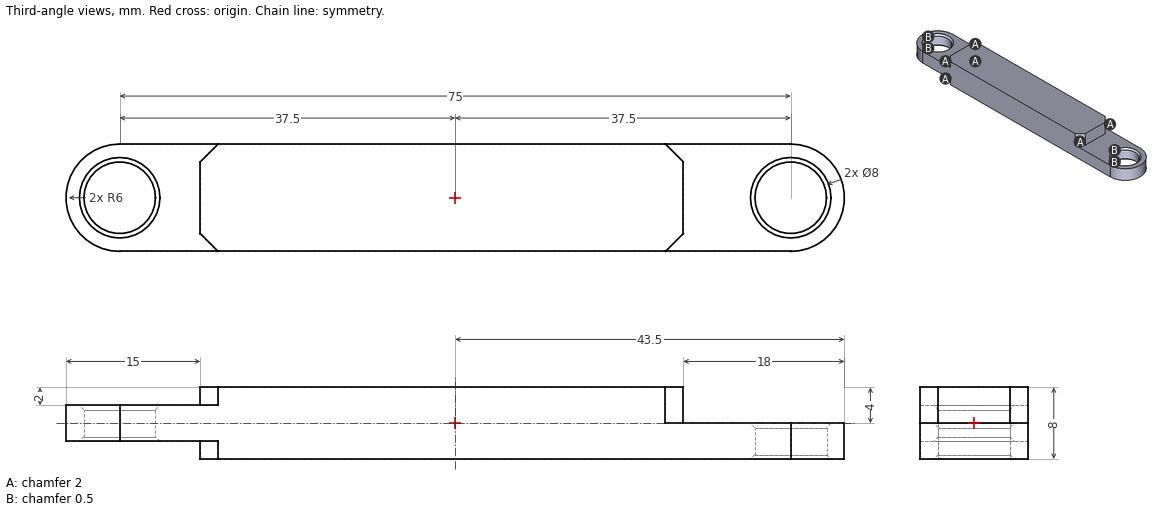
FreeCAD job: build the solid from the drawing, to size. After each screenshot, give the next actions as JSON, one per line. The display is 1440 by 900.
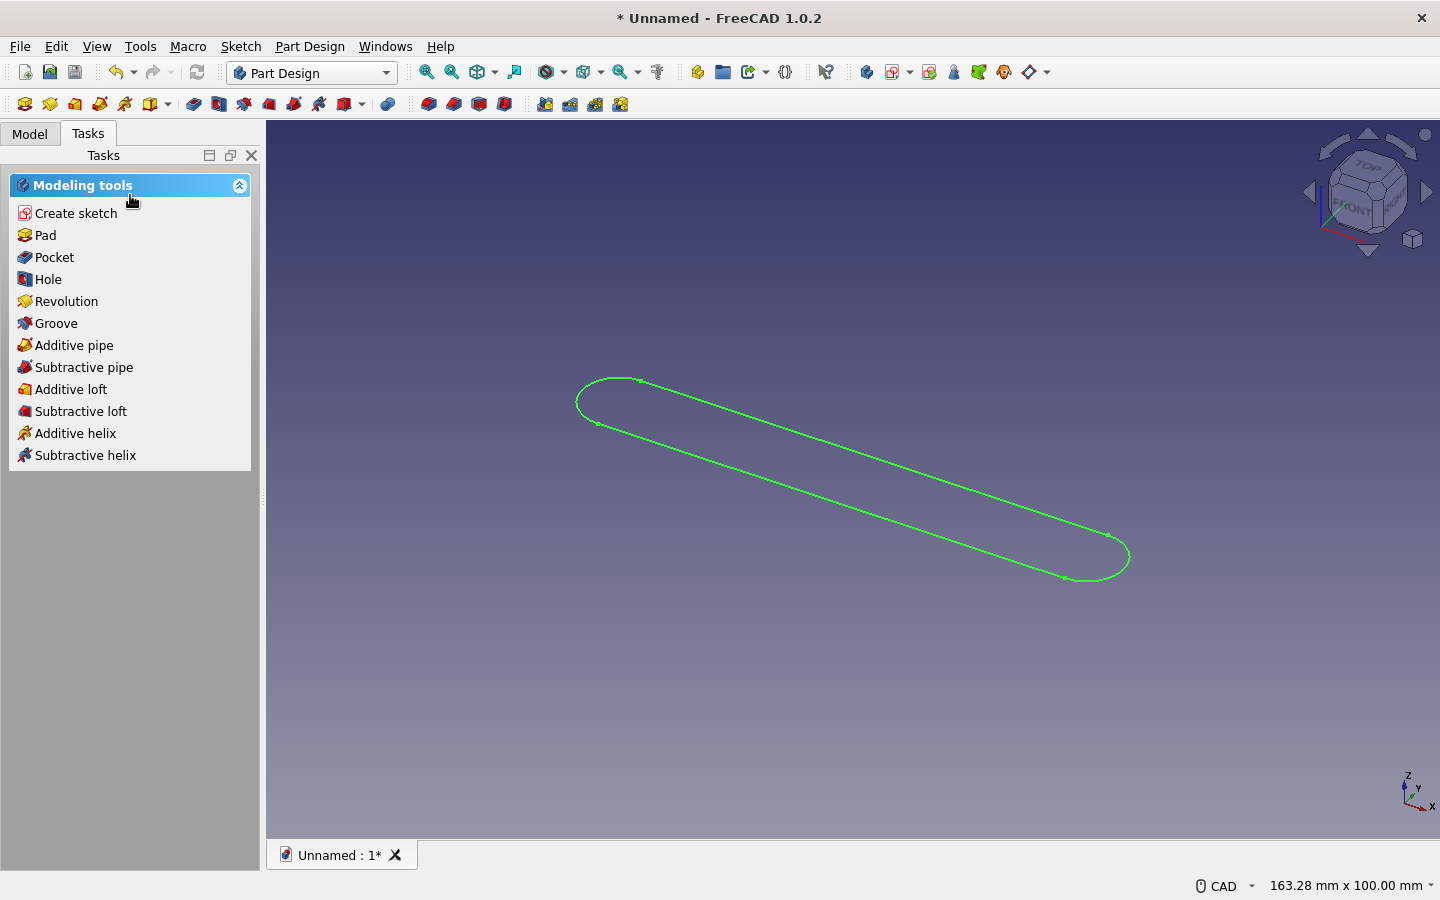
{"action": "left_click", "coordinate": [25, 104]}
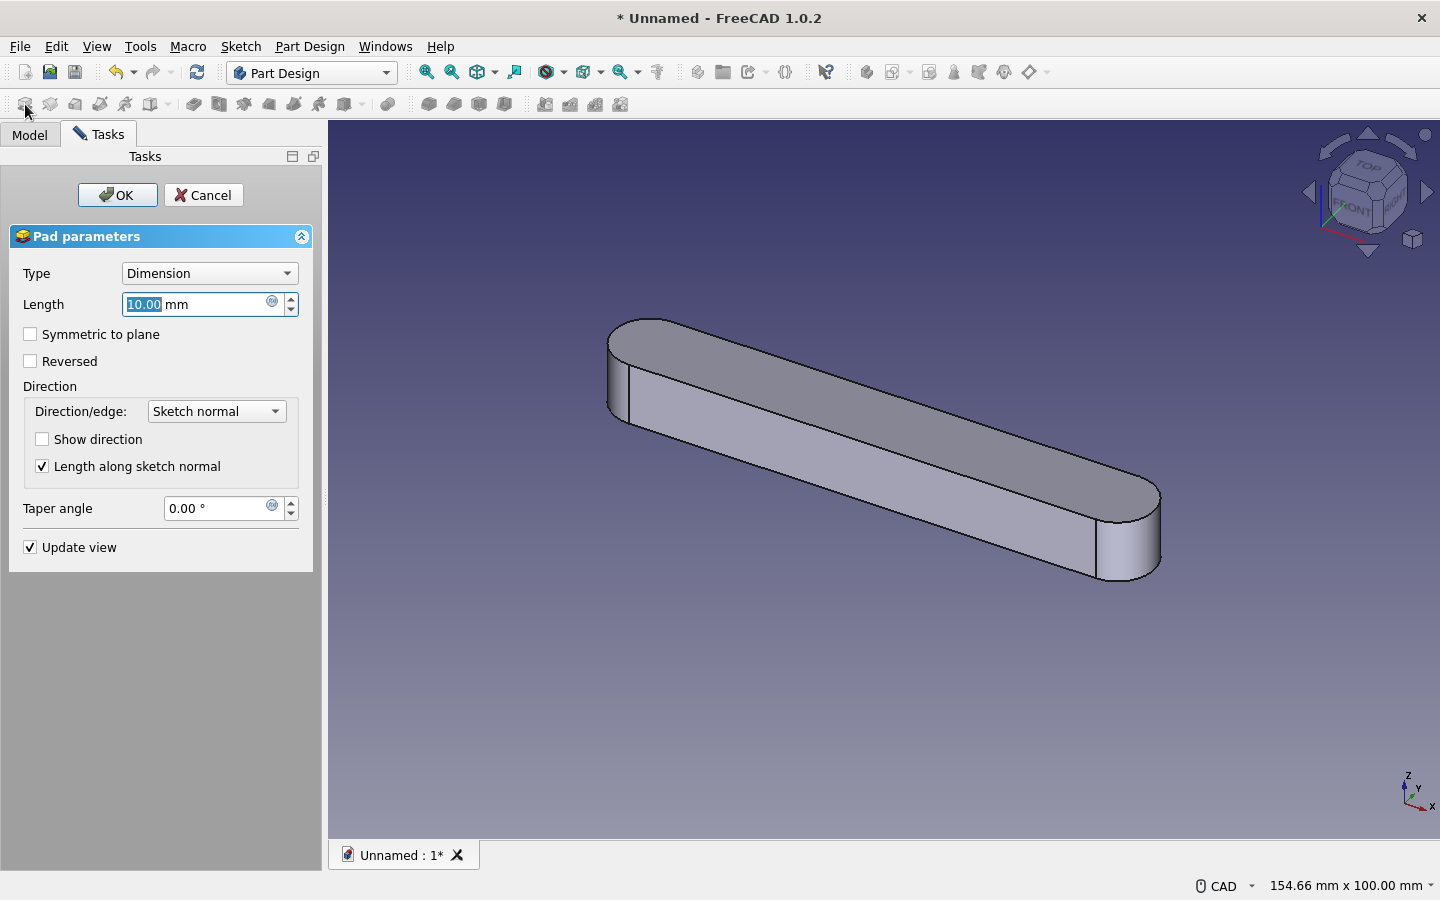
{"action": "type", "text": "8"}
{"action": "key", "text": "Tab"}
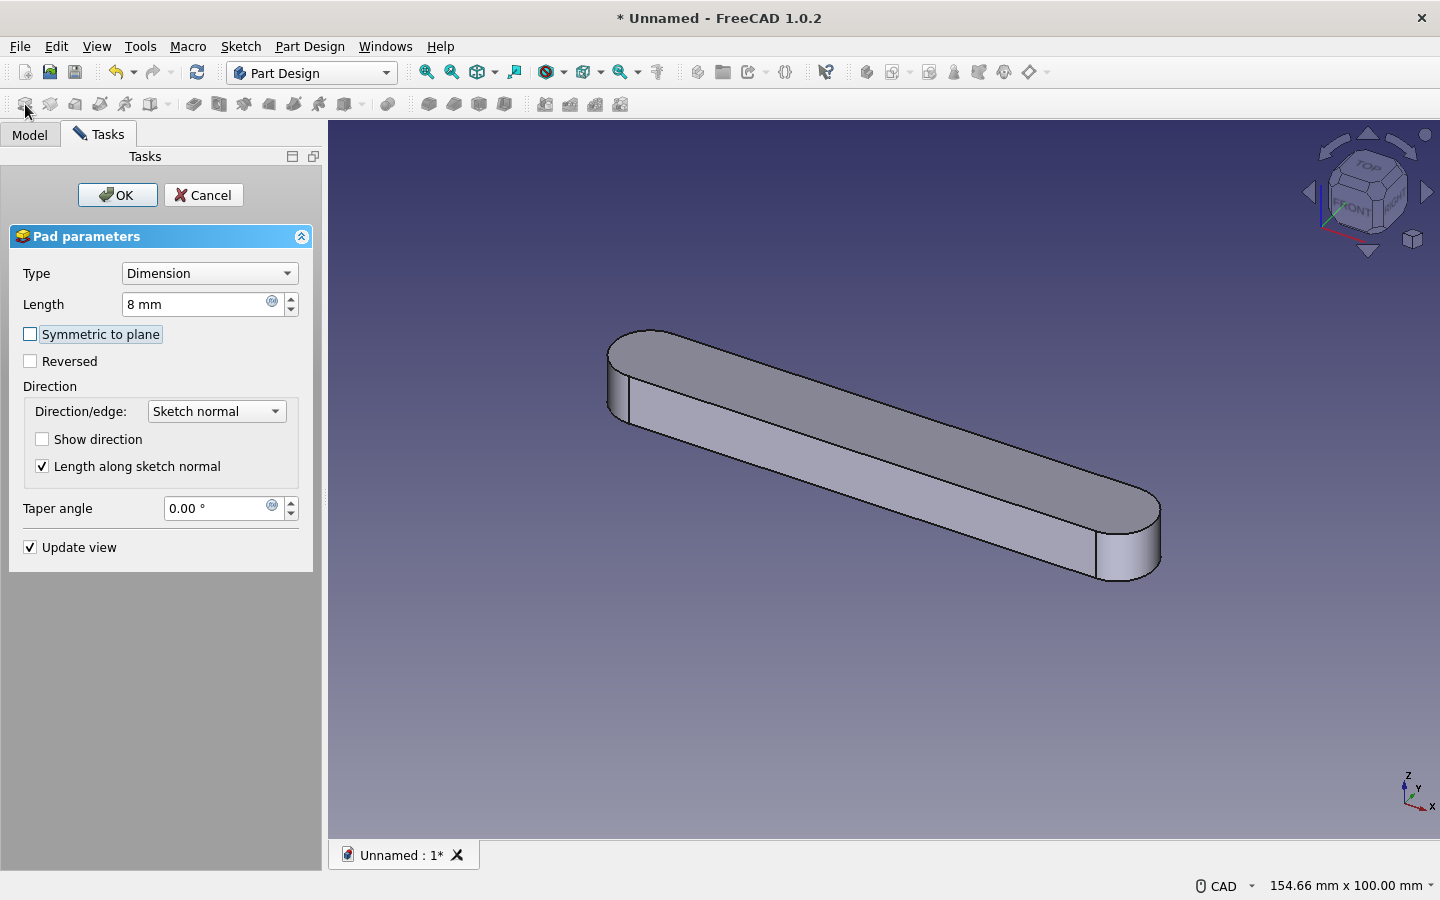
{"action": "left_click", "coordinate": [31, 334]}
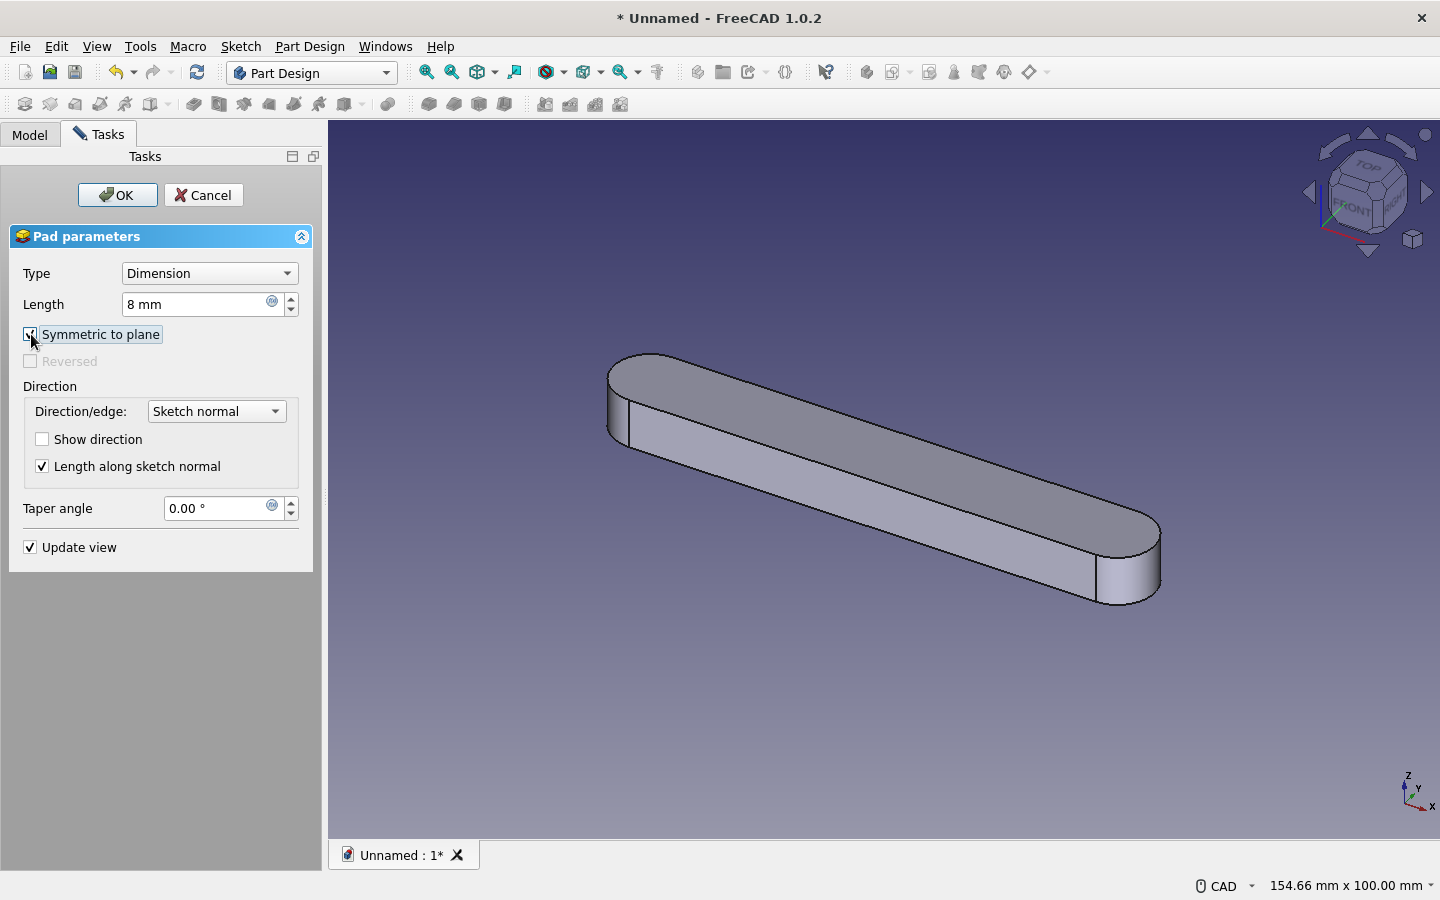
{"action": "left_click", "coordinate": [118, 195]}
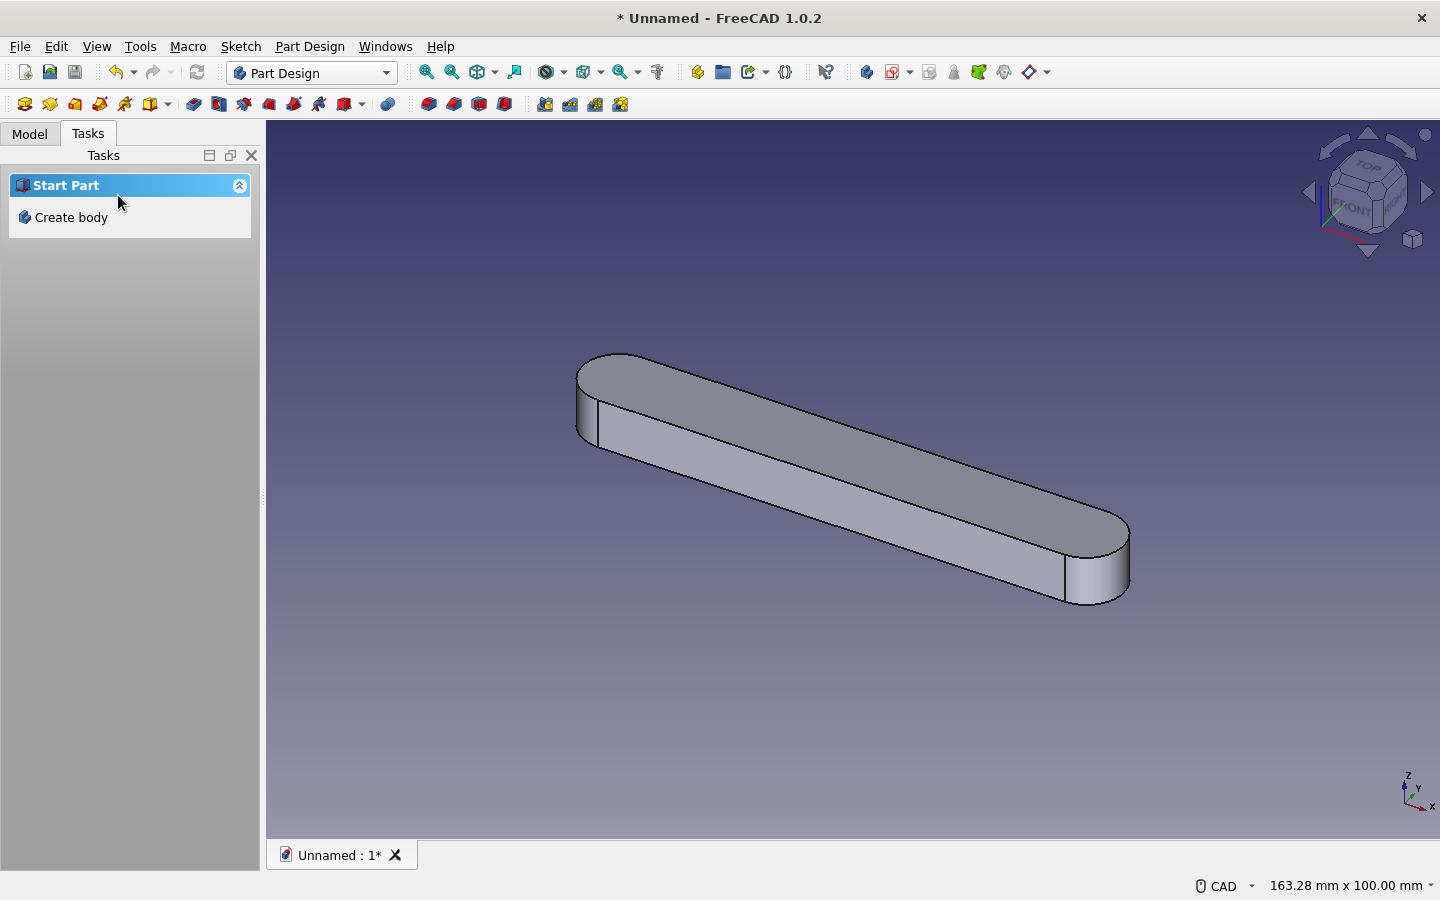
{"action": "left_click", "coordinate": [1085, 532]}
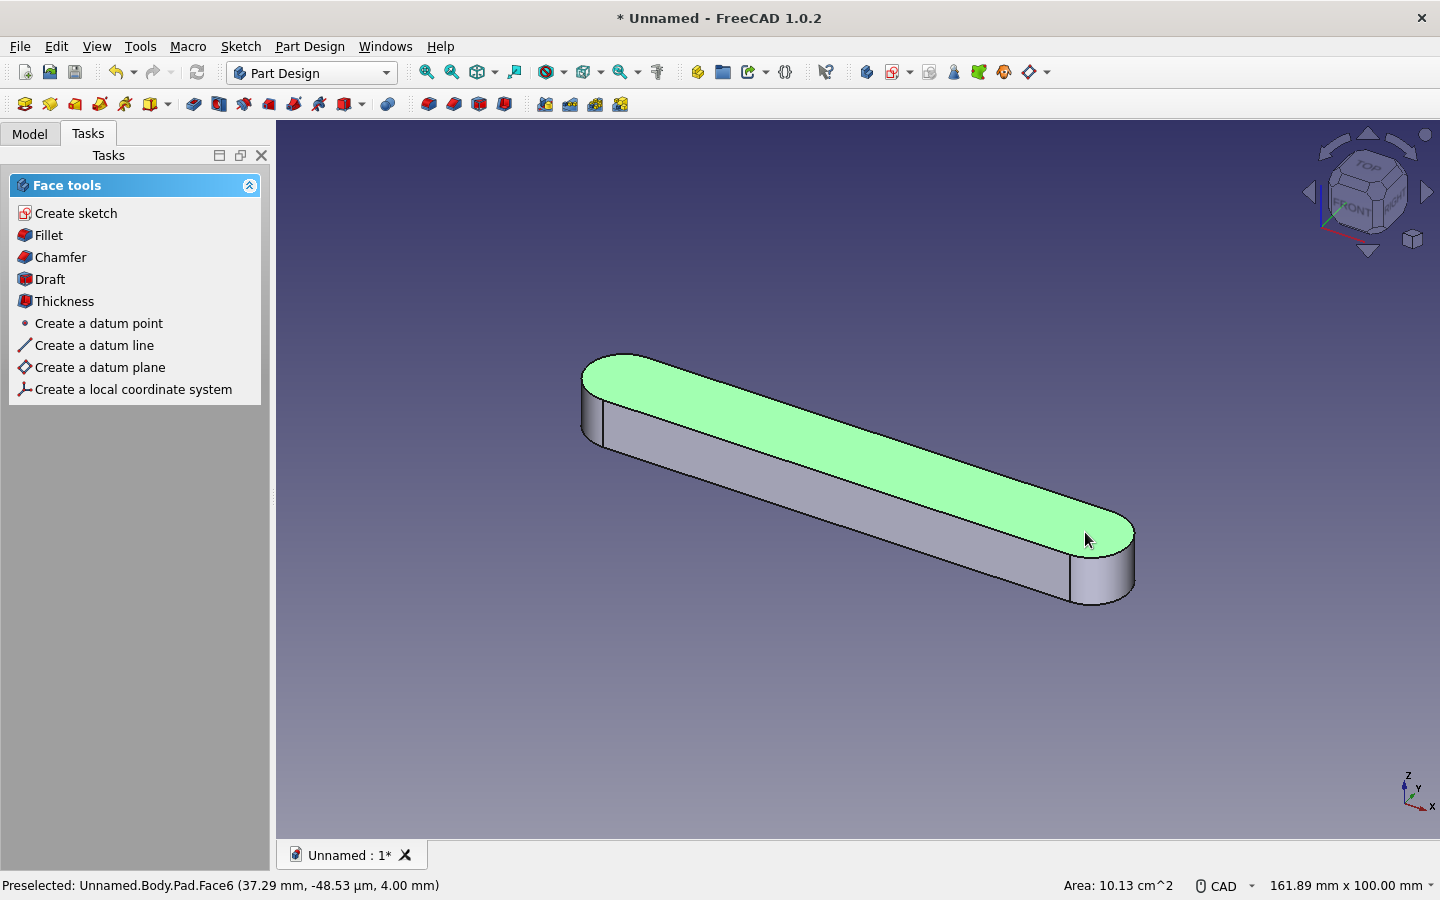
{"action": "left_click", "coordinate": [892, 72]}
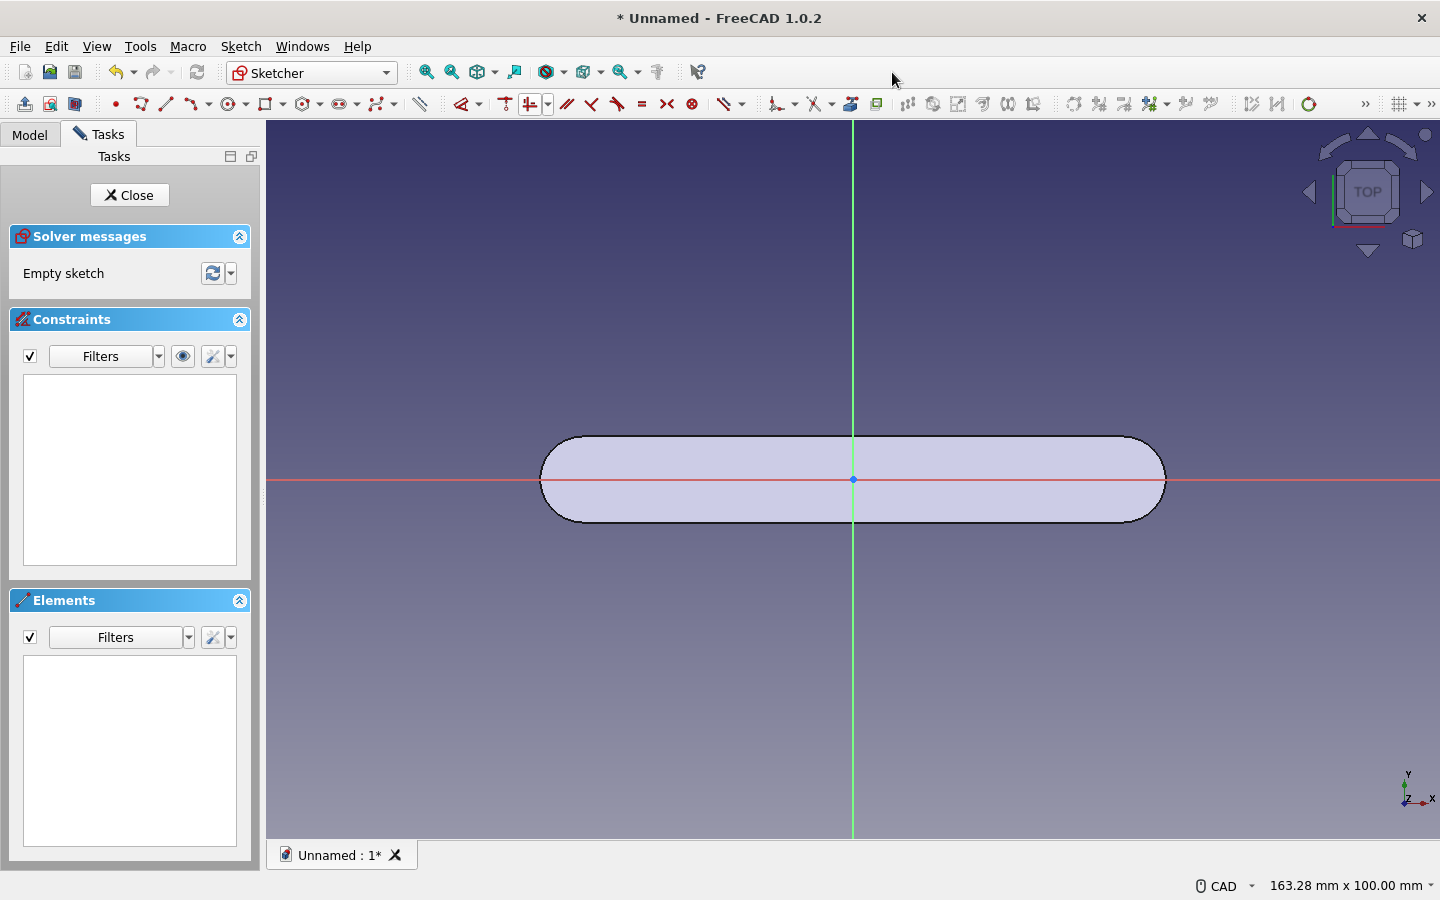
{"action": "key", "text": "g c"}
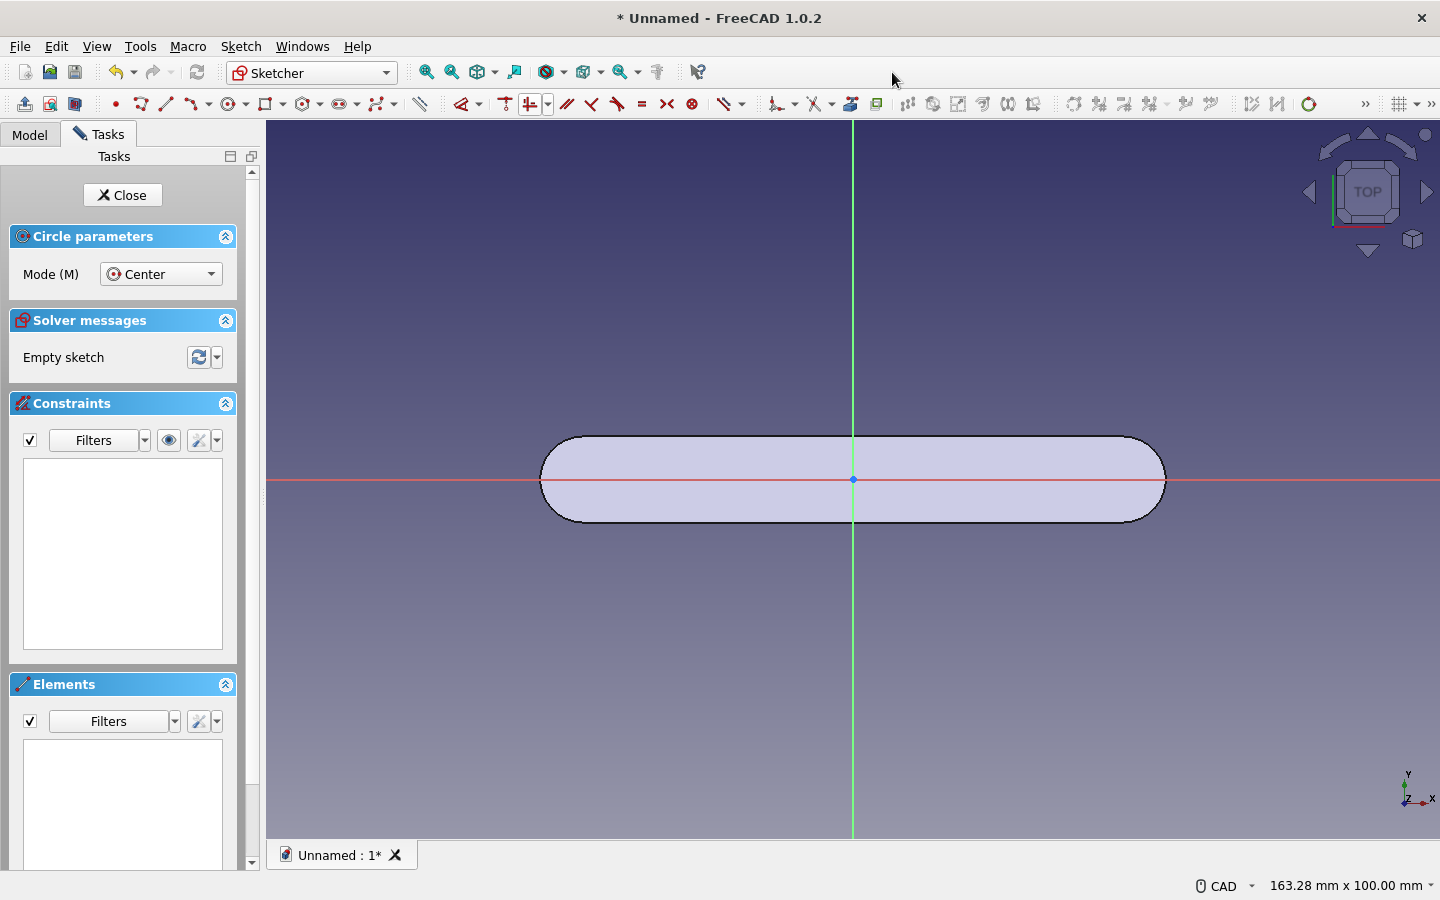
{"action": "left_click", "coordinate": [1123, 480]}
{"action": "left_click", "coordinate": [1143, 459]}